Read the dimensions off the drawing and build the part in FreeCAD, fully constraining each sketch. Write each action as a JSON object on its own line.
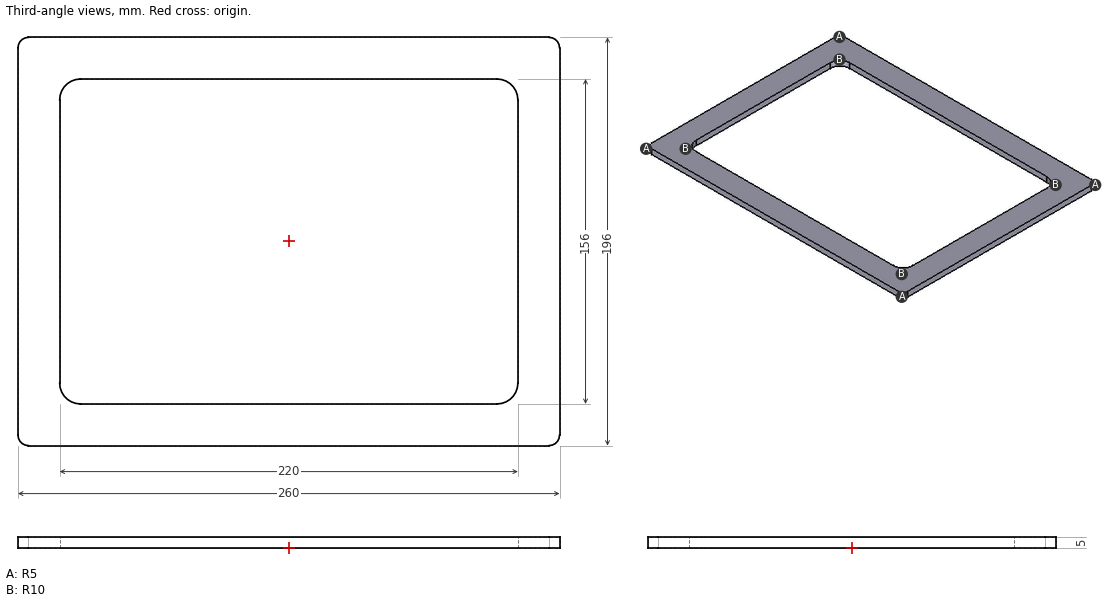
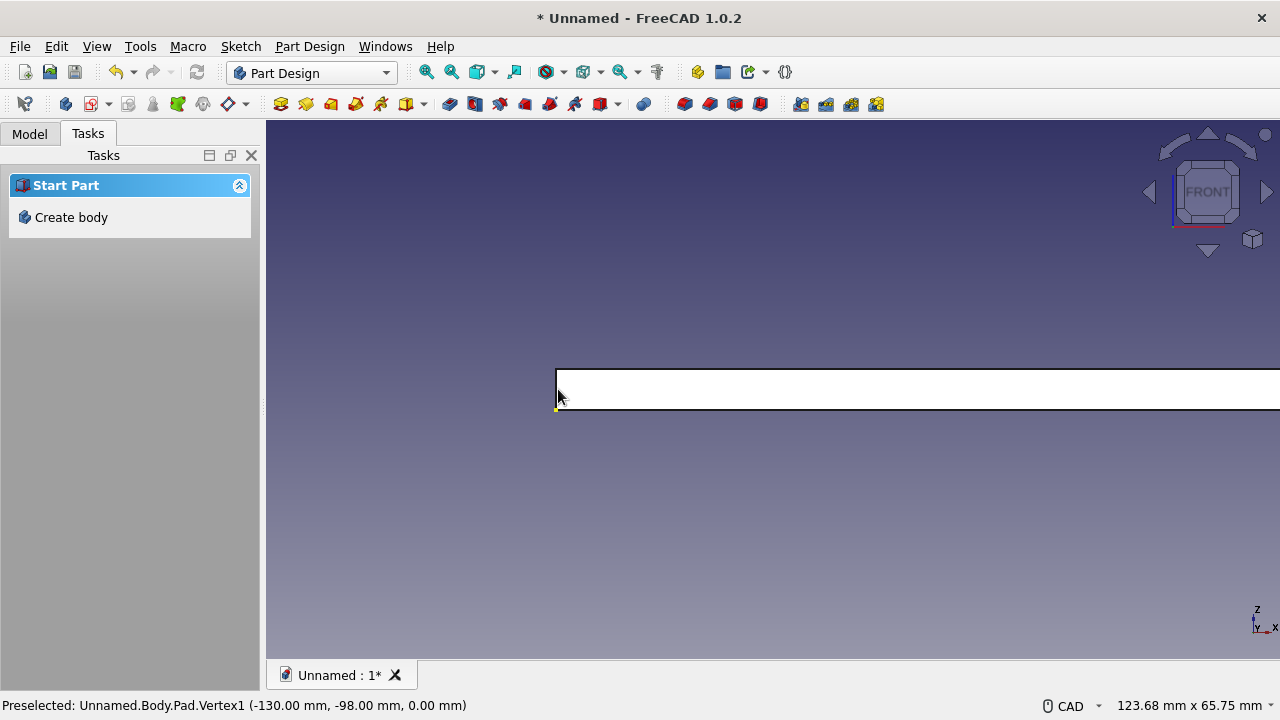
{"action": "left_click", "coordinate": [556, 389]}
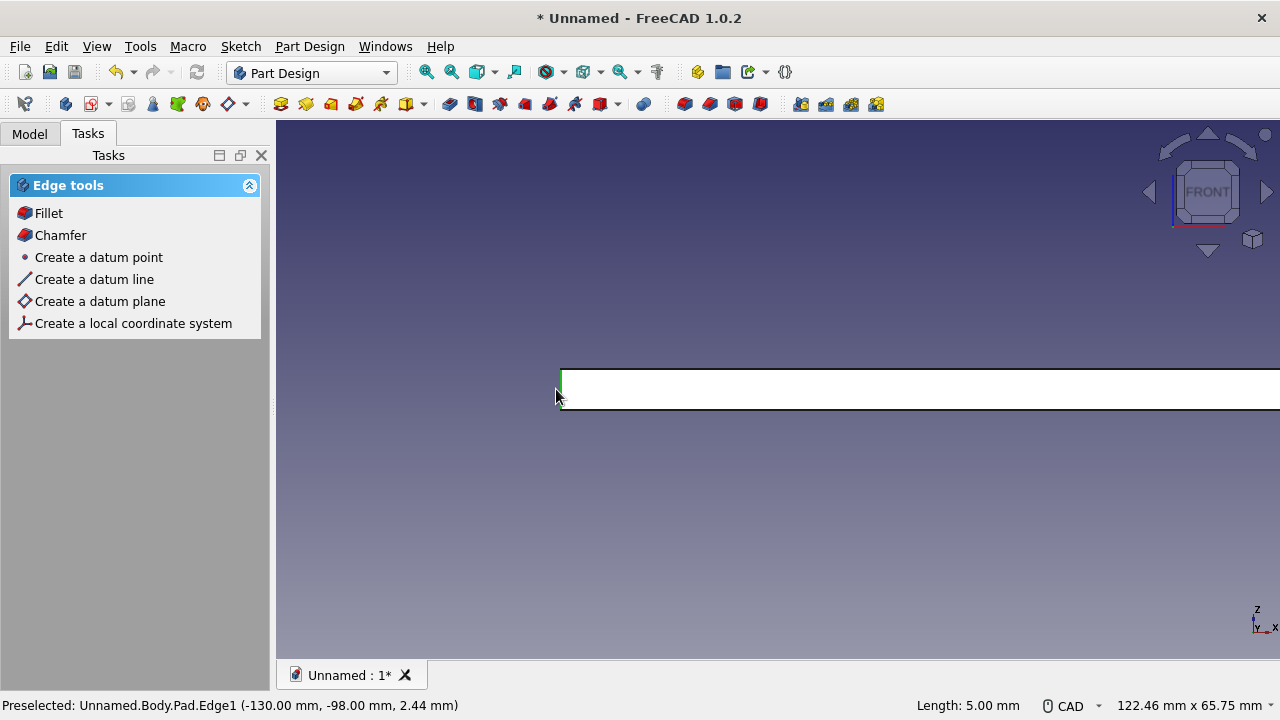
{"action": "left_click", "coordinate": [427, 72]}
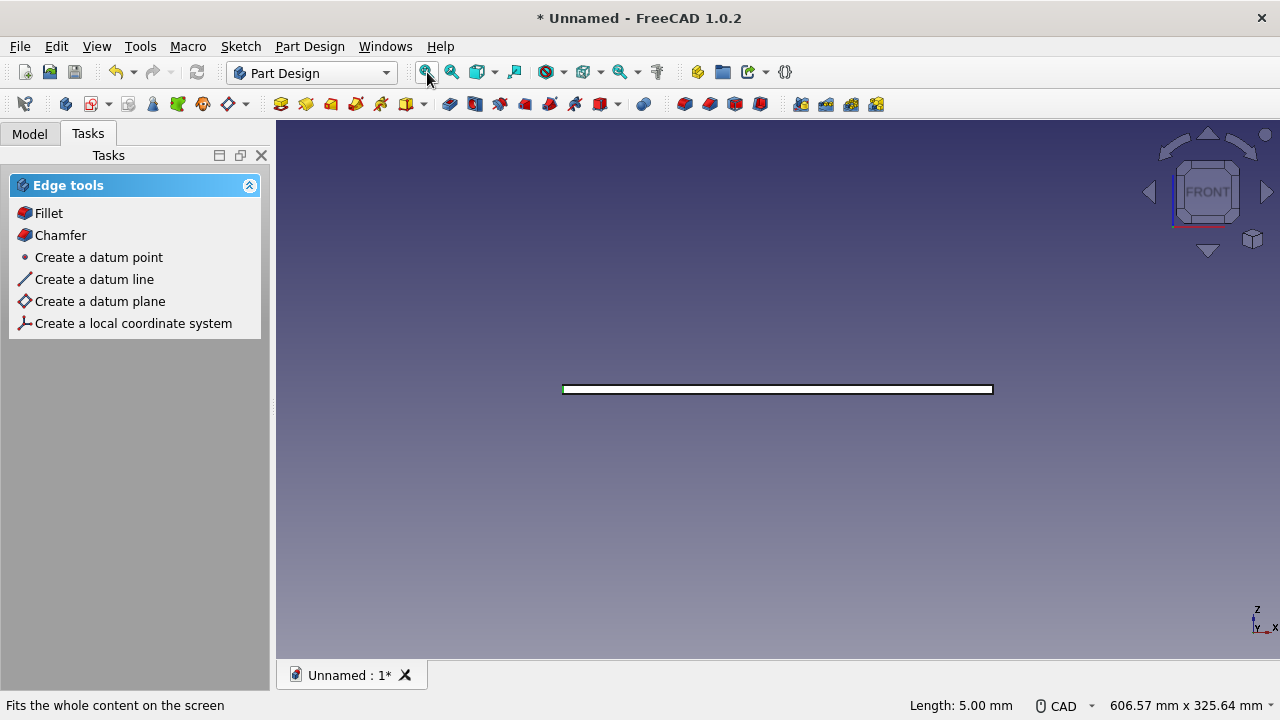
{"action": "key", "text": "3"}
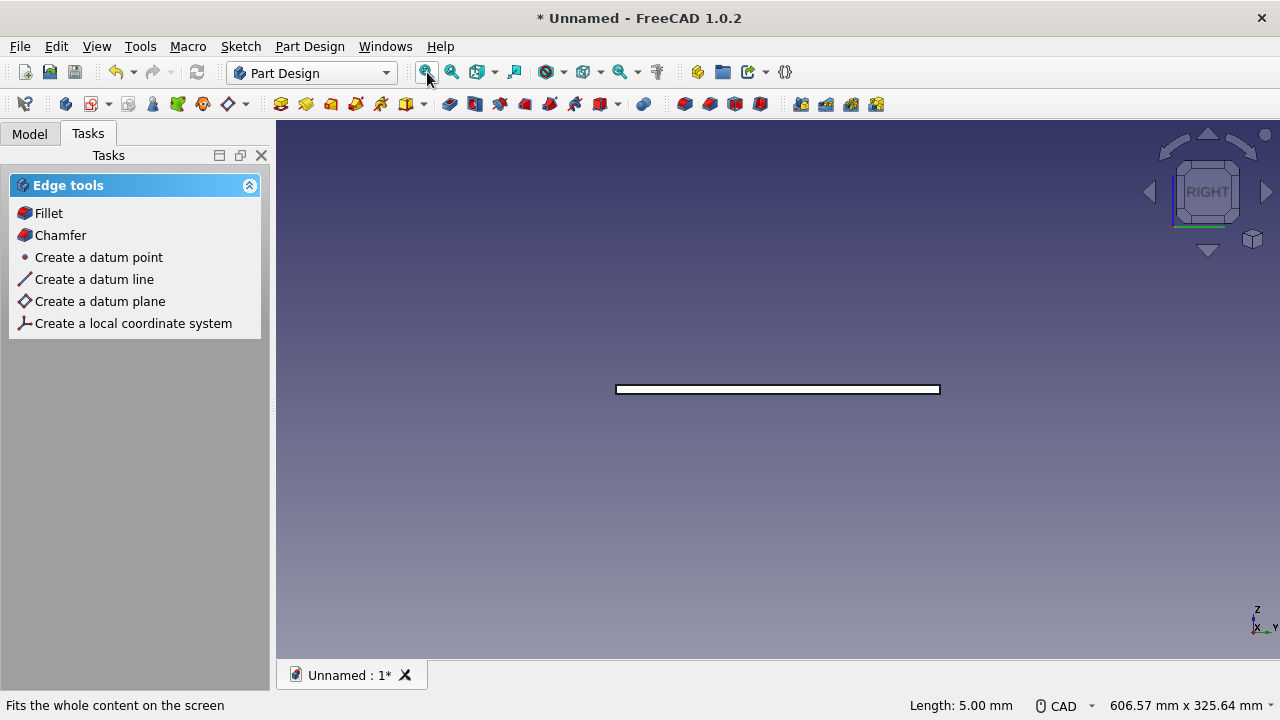
{"action": "key", "text": "v f"}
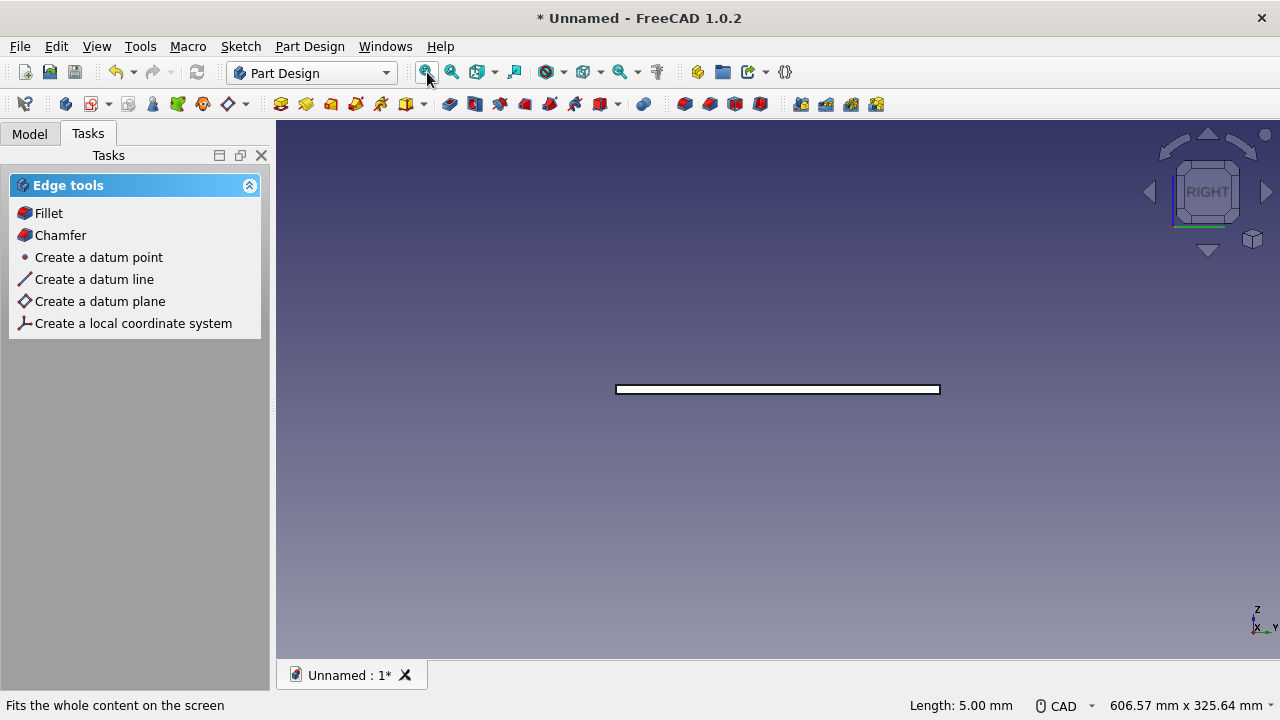
{"action": "scroll", "coordinate": [940, 388], "scroll_direction": "up", "scroll_amount": 8}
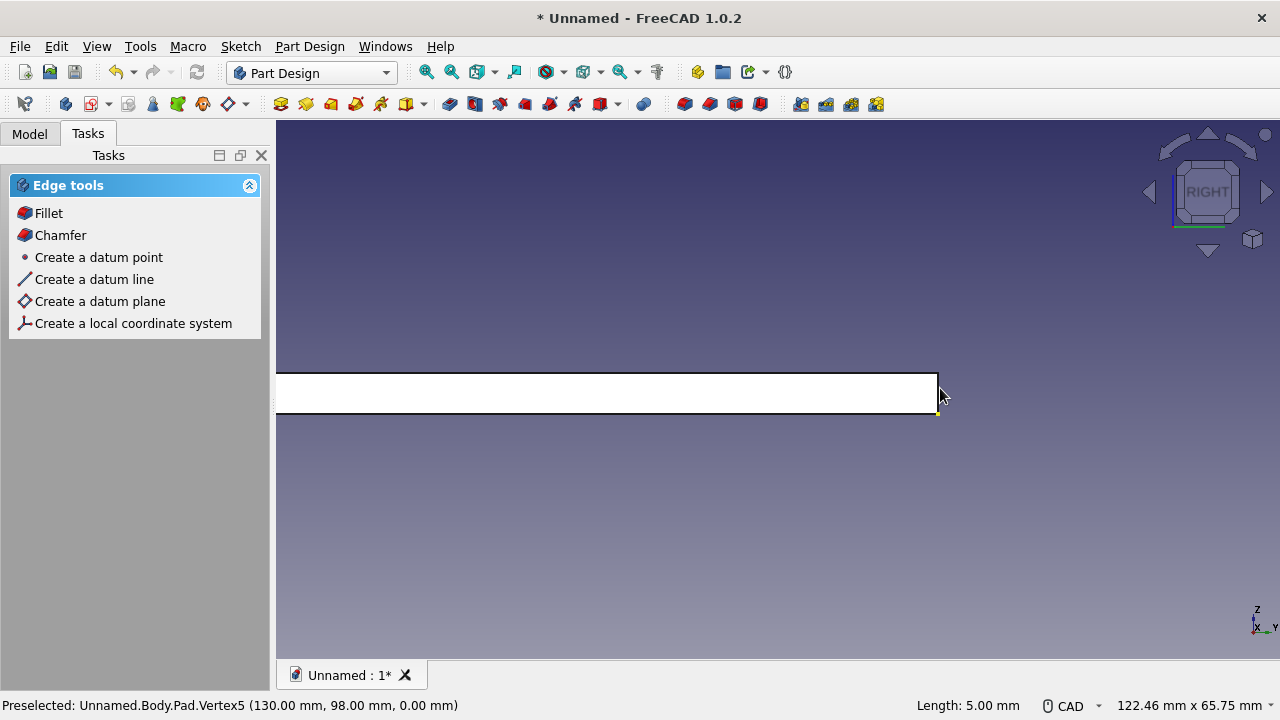
{"action": "left_click", "coordinate": [938, 392], "text": "ctrl"}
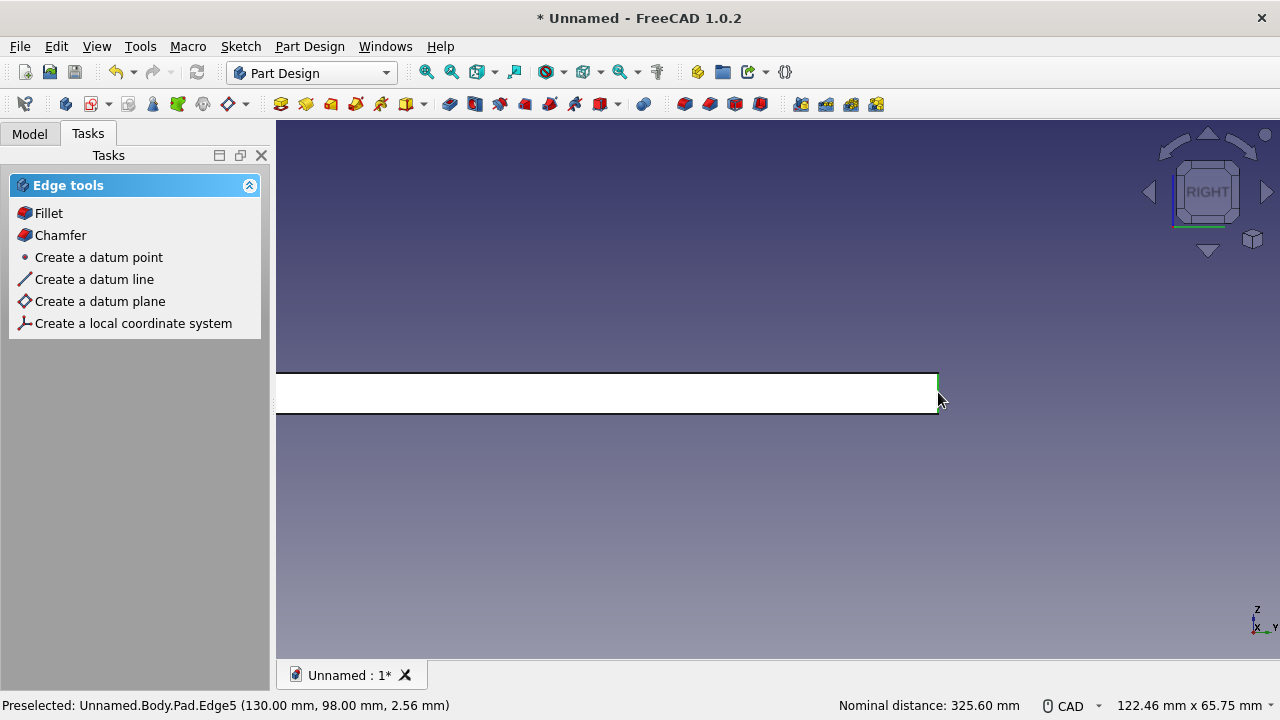
{"action": "key", "text": "v f"}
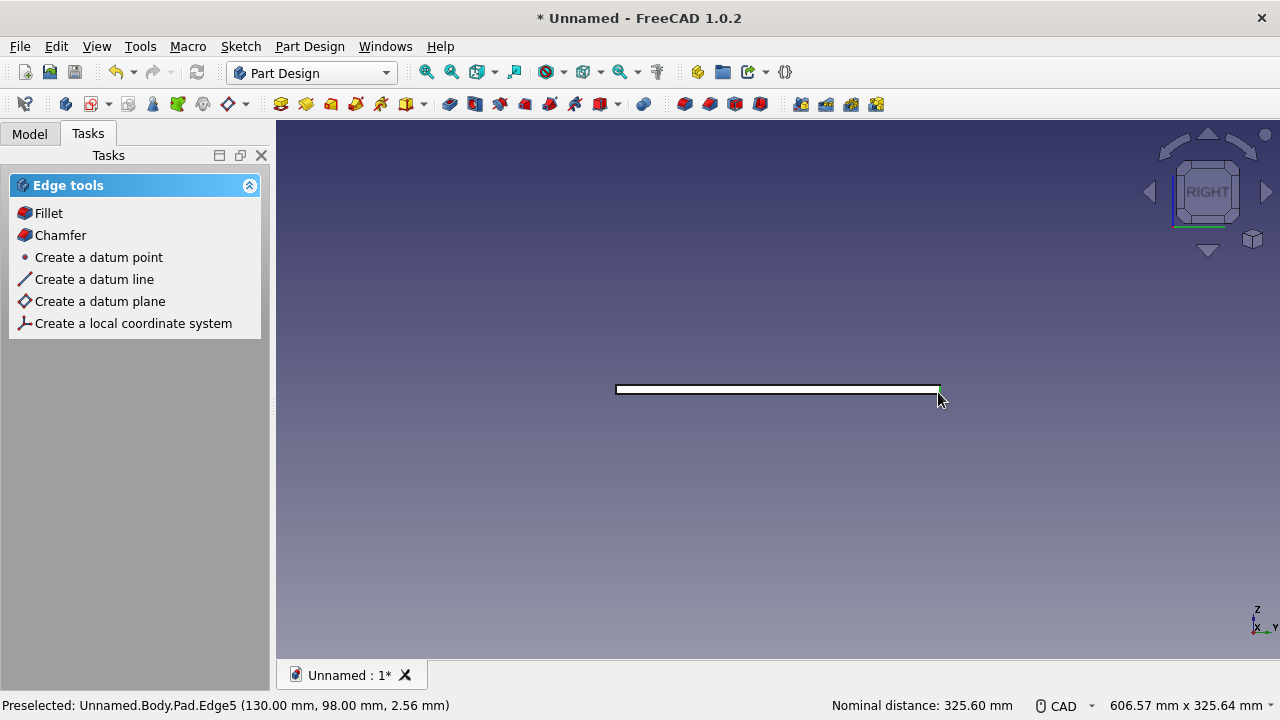
{"action": "key", "text": "5"}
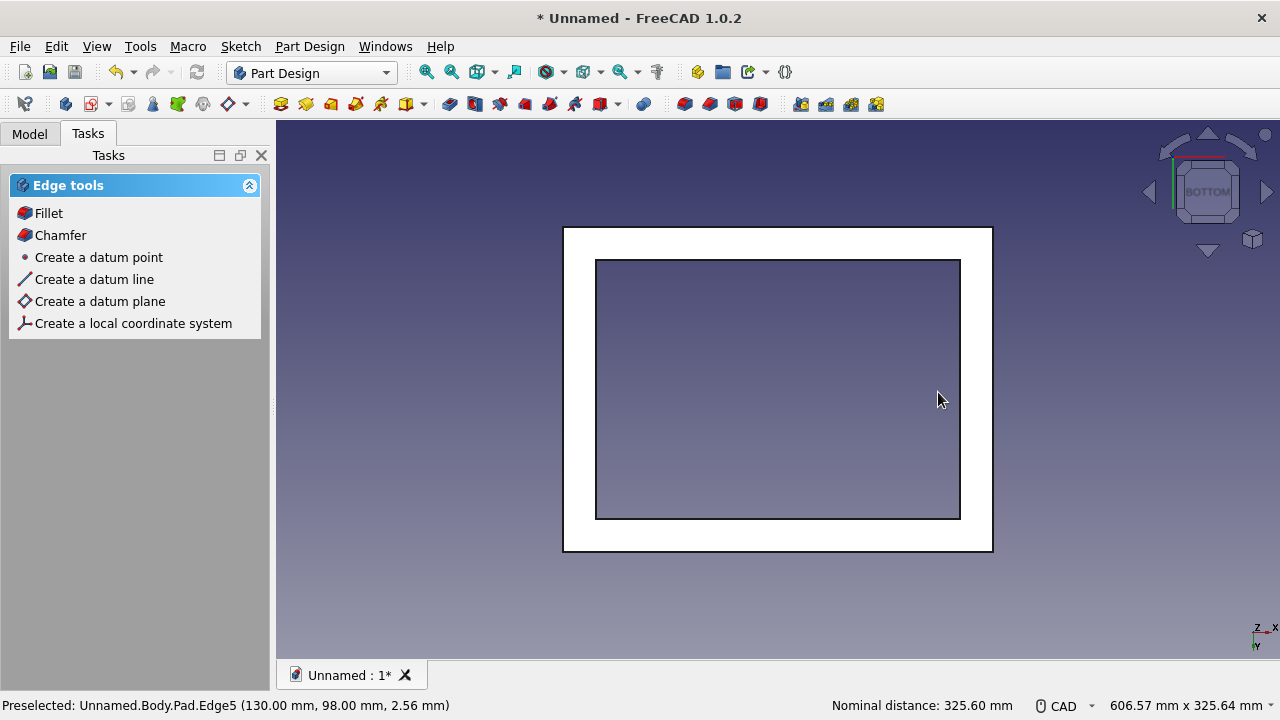
{"action": "scroll", "coordinate": [563, 551], "scroll_direction": "up", "scroll_amount": 8}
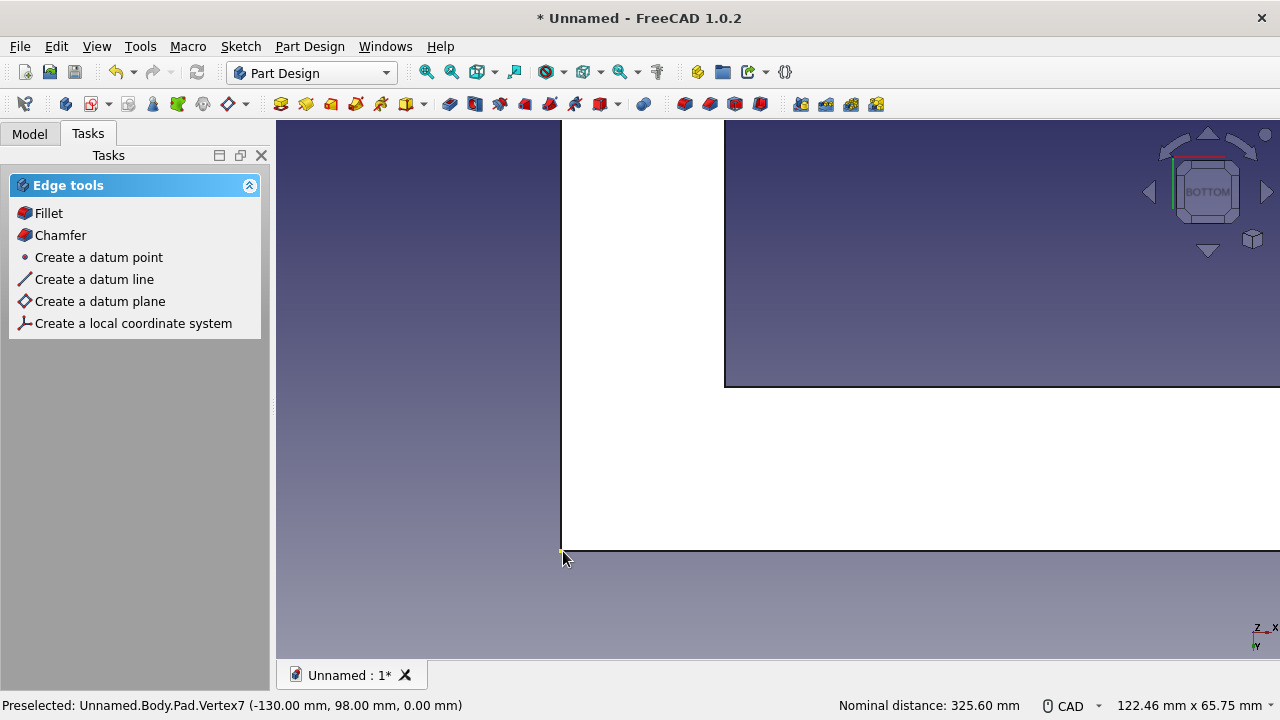
{"action": "key", "text": "v f"}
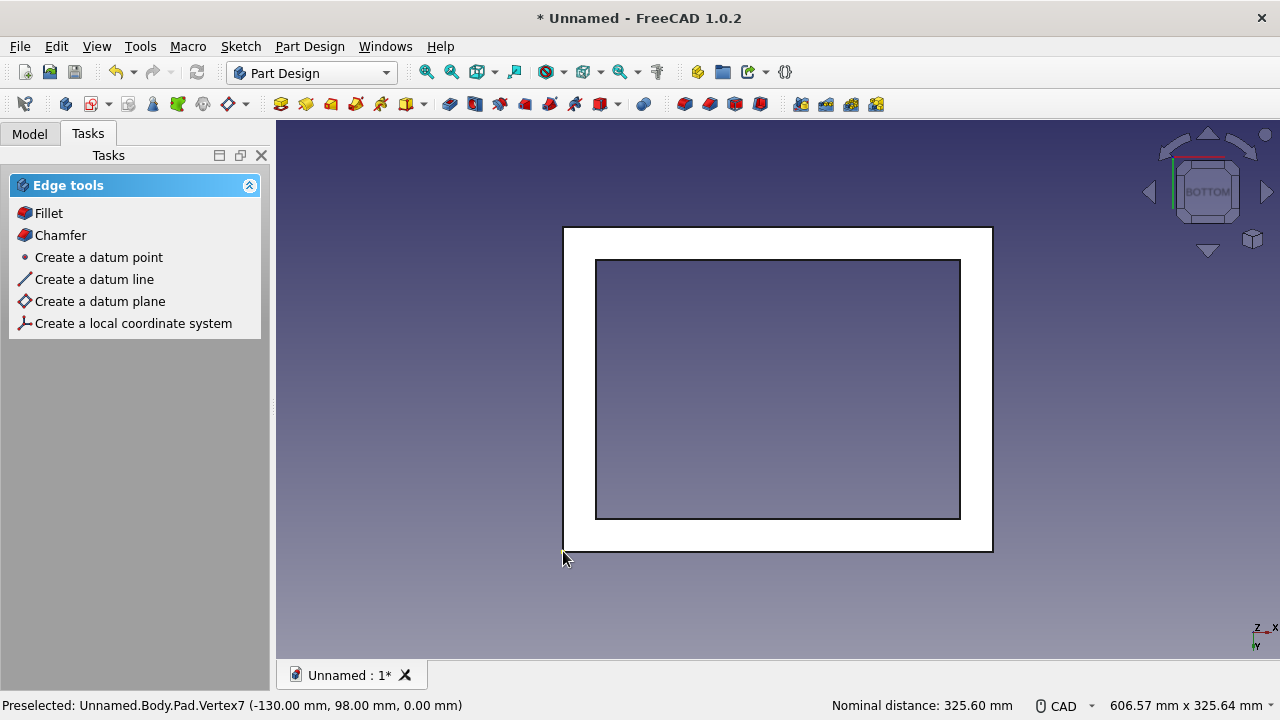
{"action": "key", "text": "4"}